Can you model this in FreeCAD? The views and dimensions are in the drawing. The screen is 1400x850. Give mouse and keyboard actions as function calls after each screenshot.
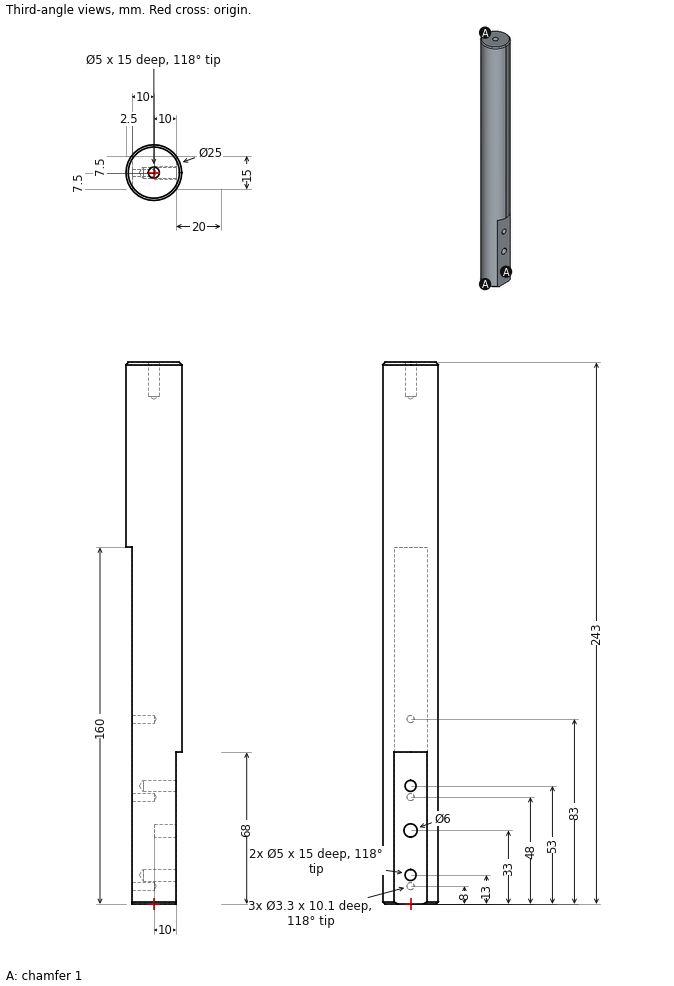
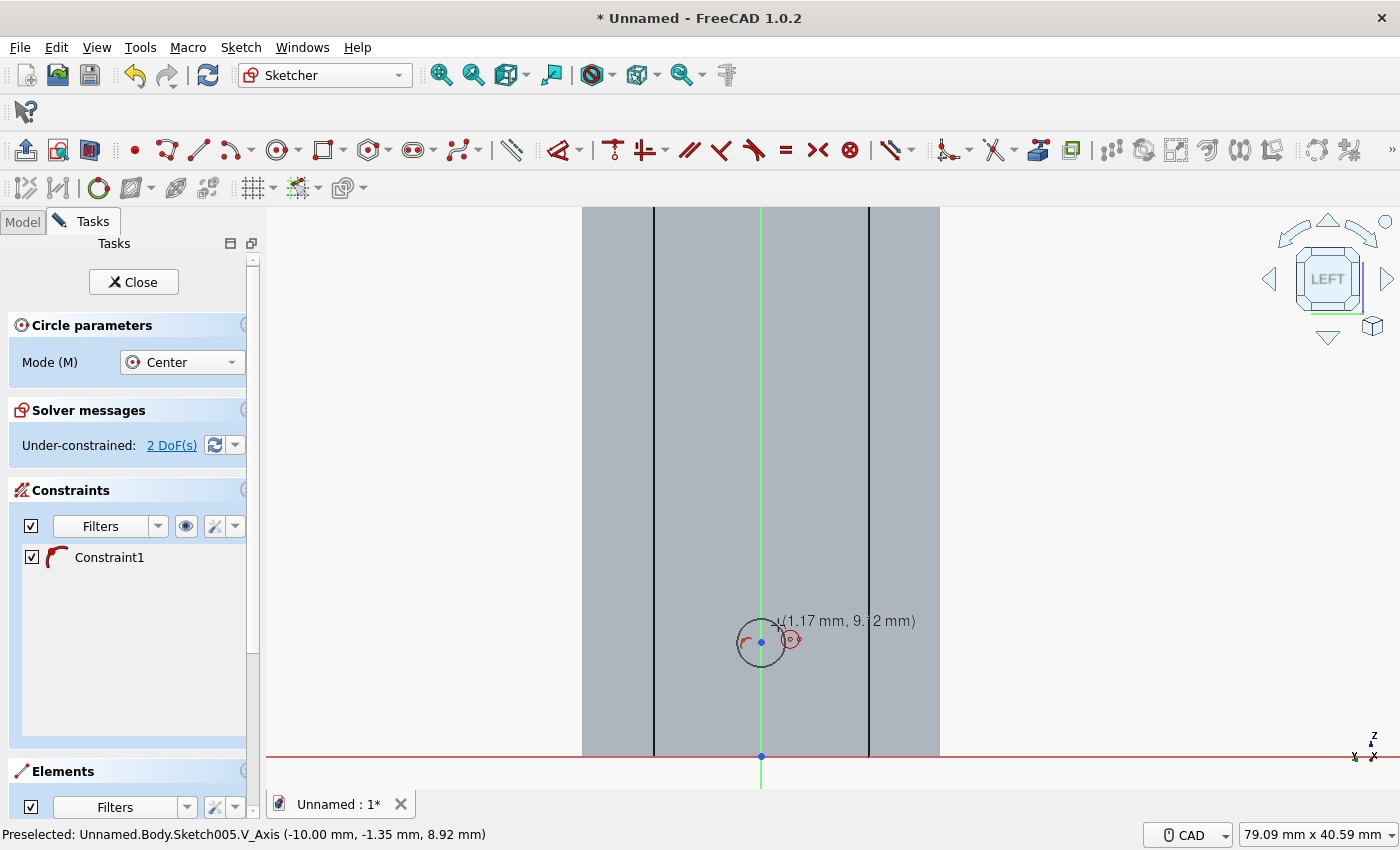
scroll(766, 648, down, 6)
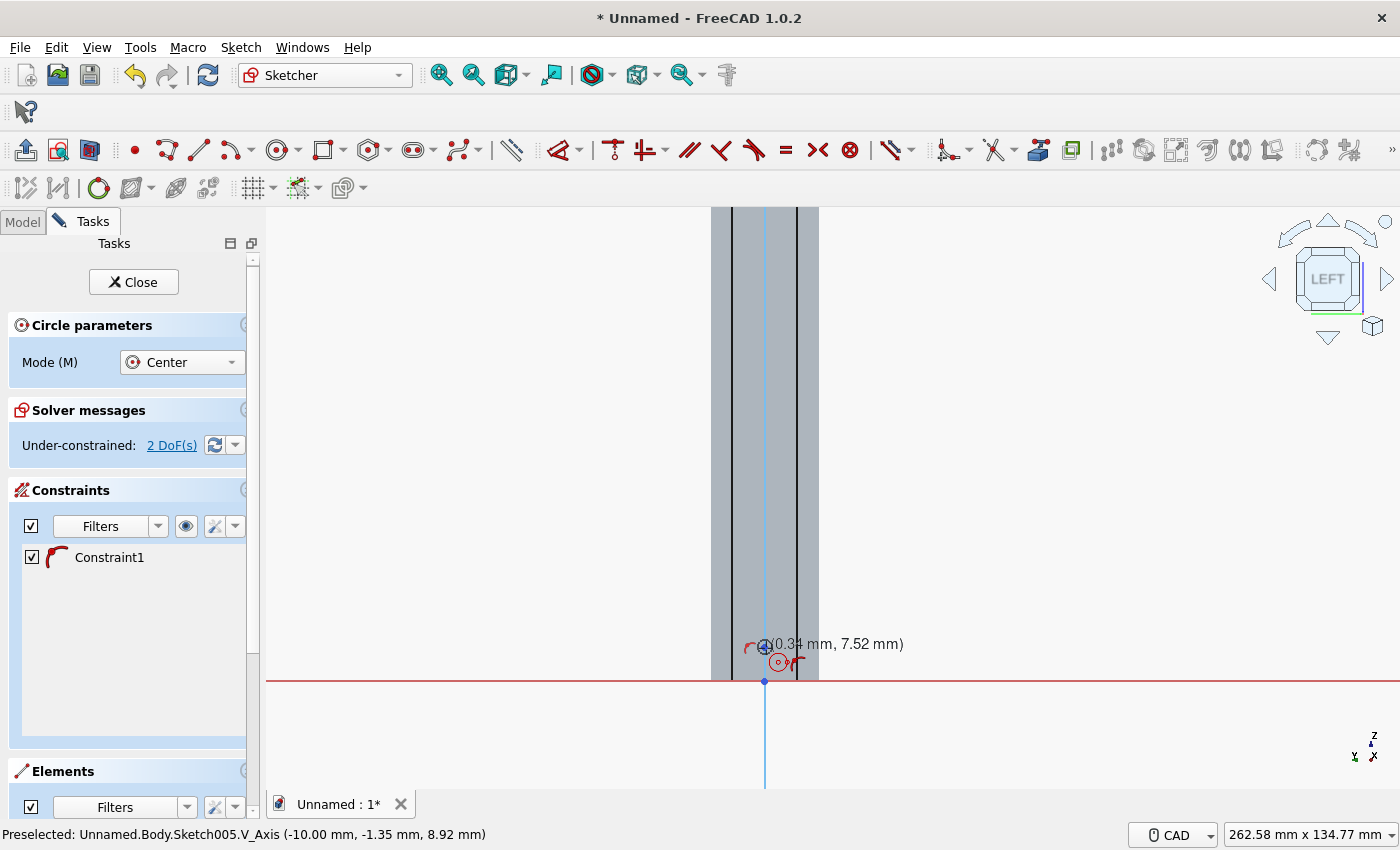
scroll(765, 323, up, 6)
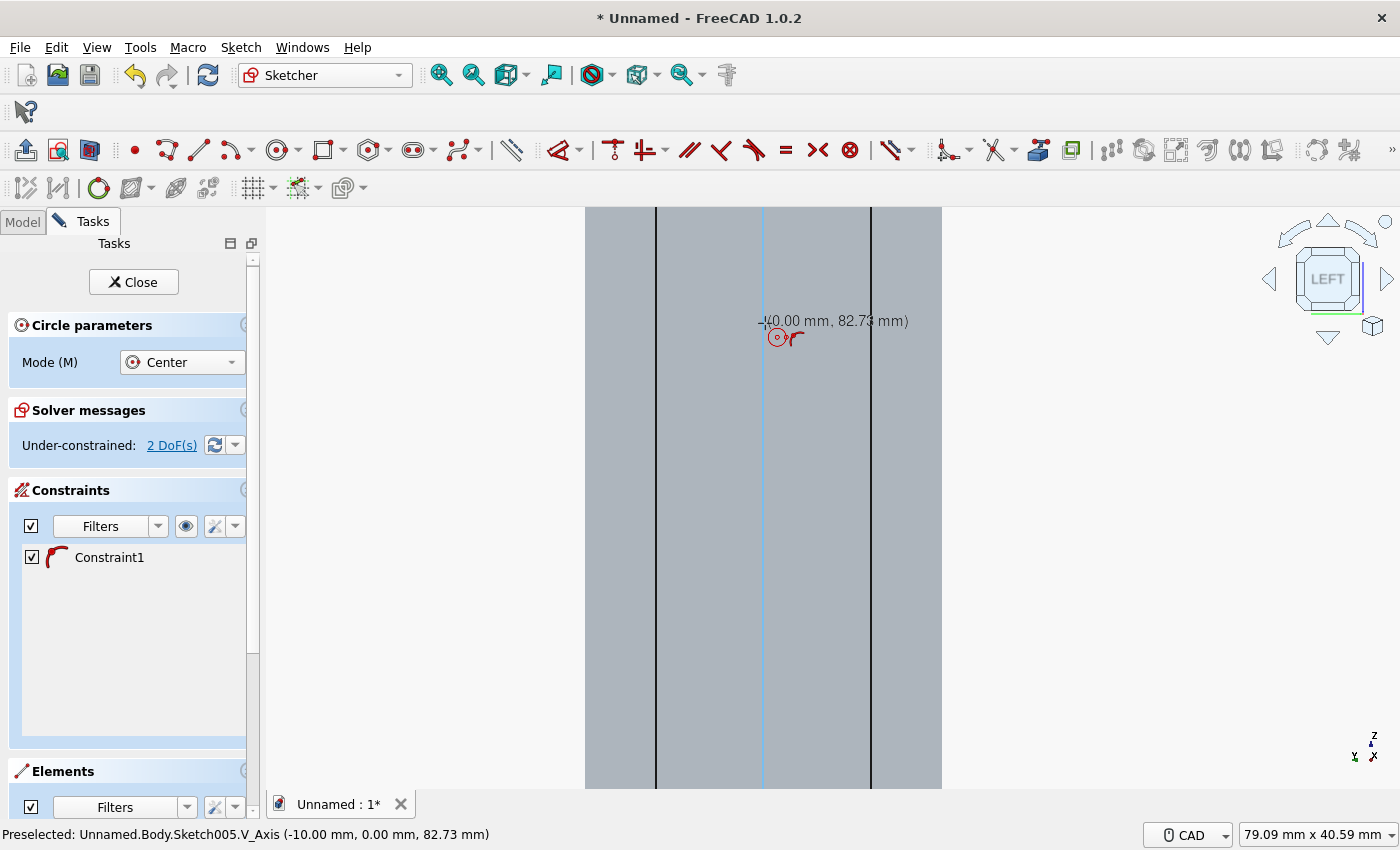
click(763, 322)
click(780, 305)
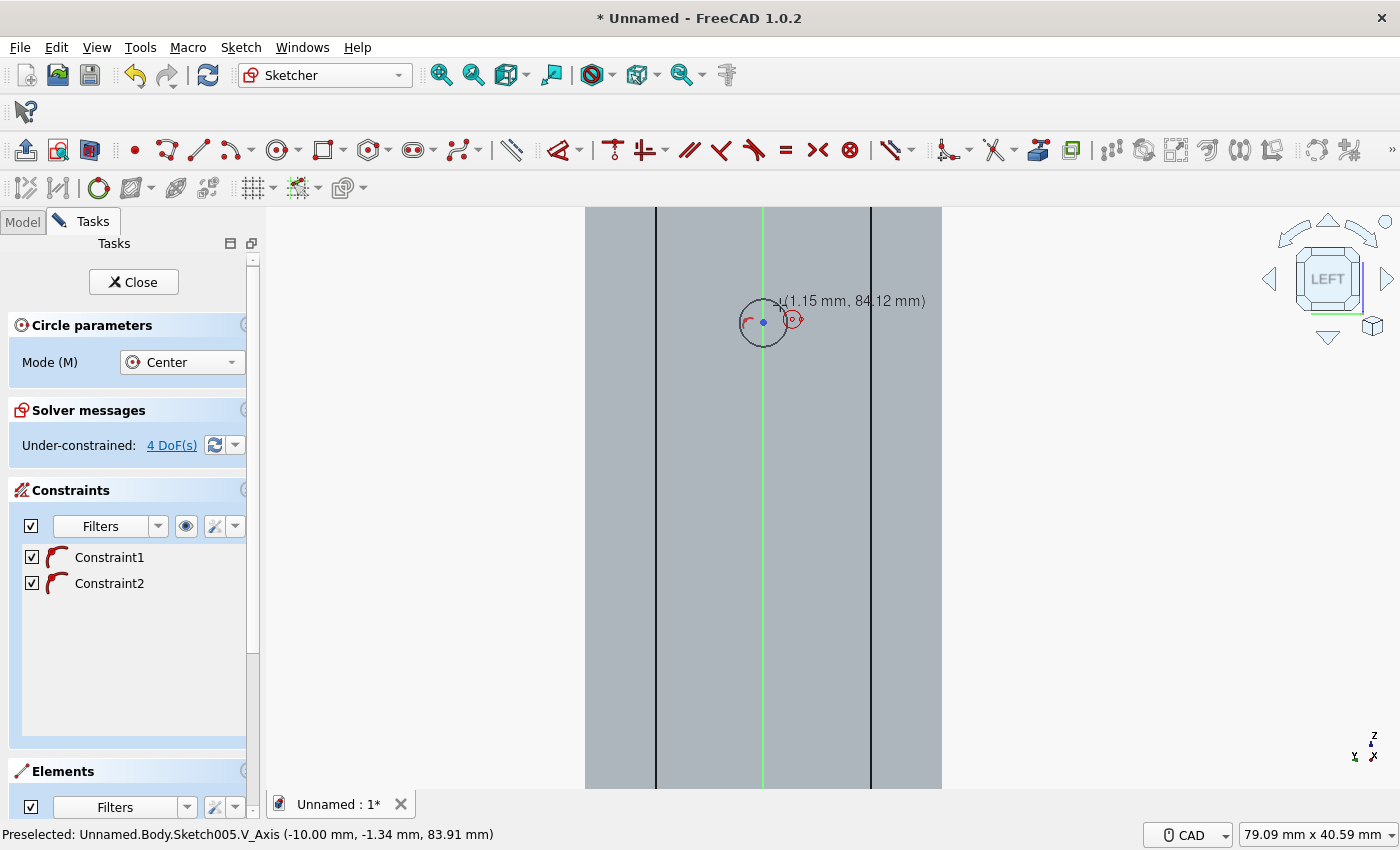
scroll(765, 322, down, 6)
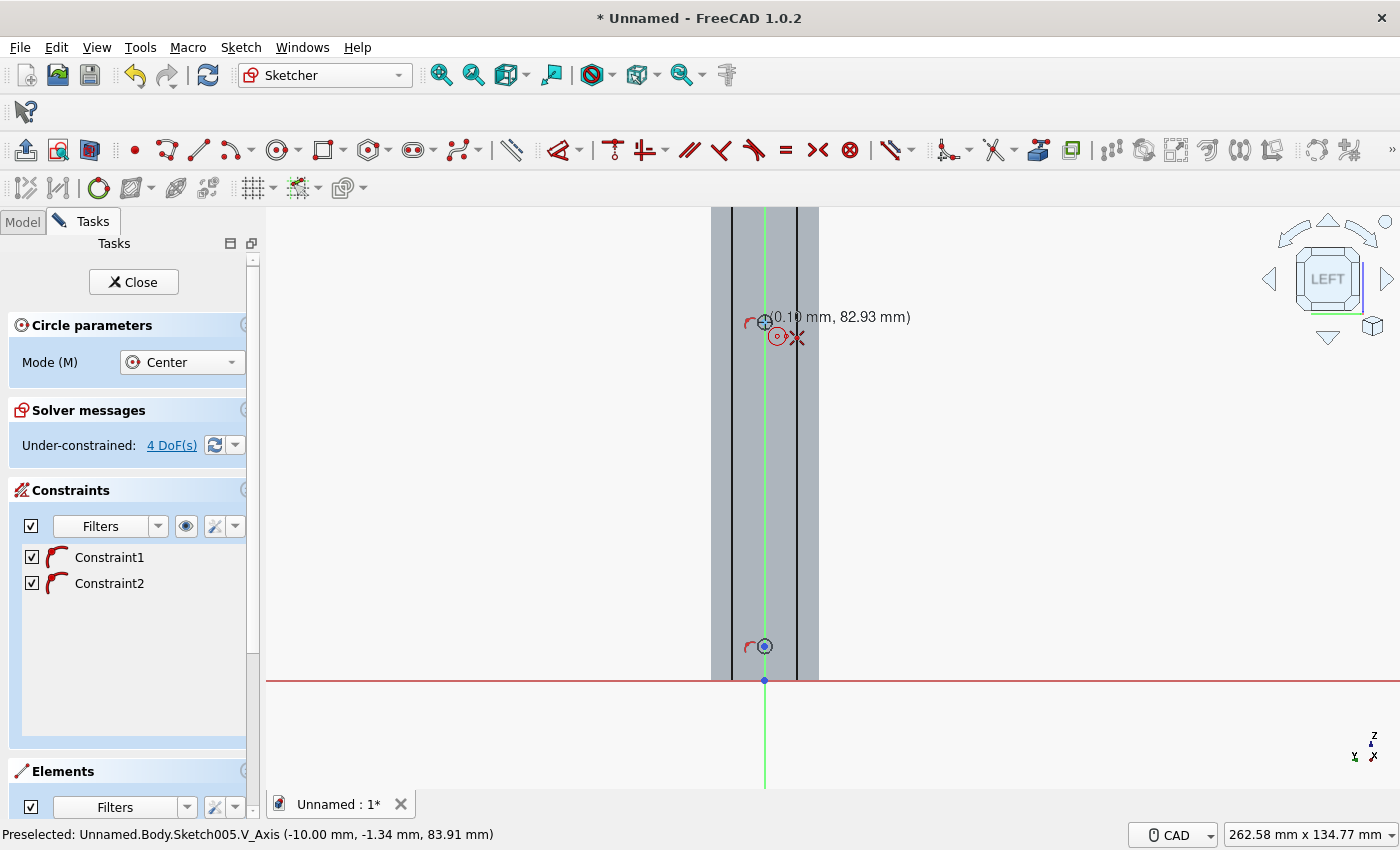
scroll(765, 473, up, 6)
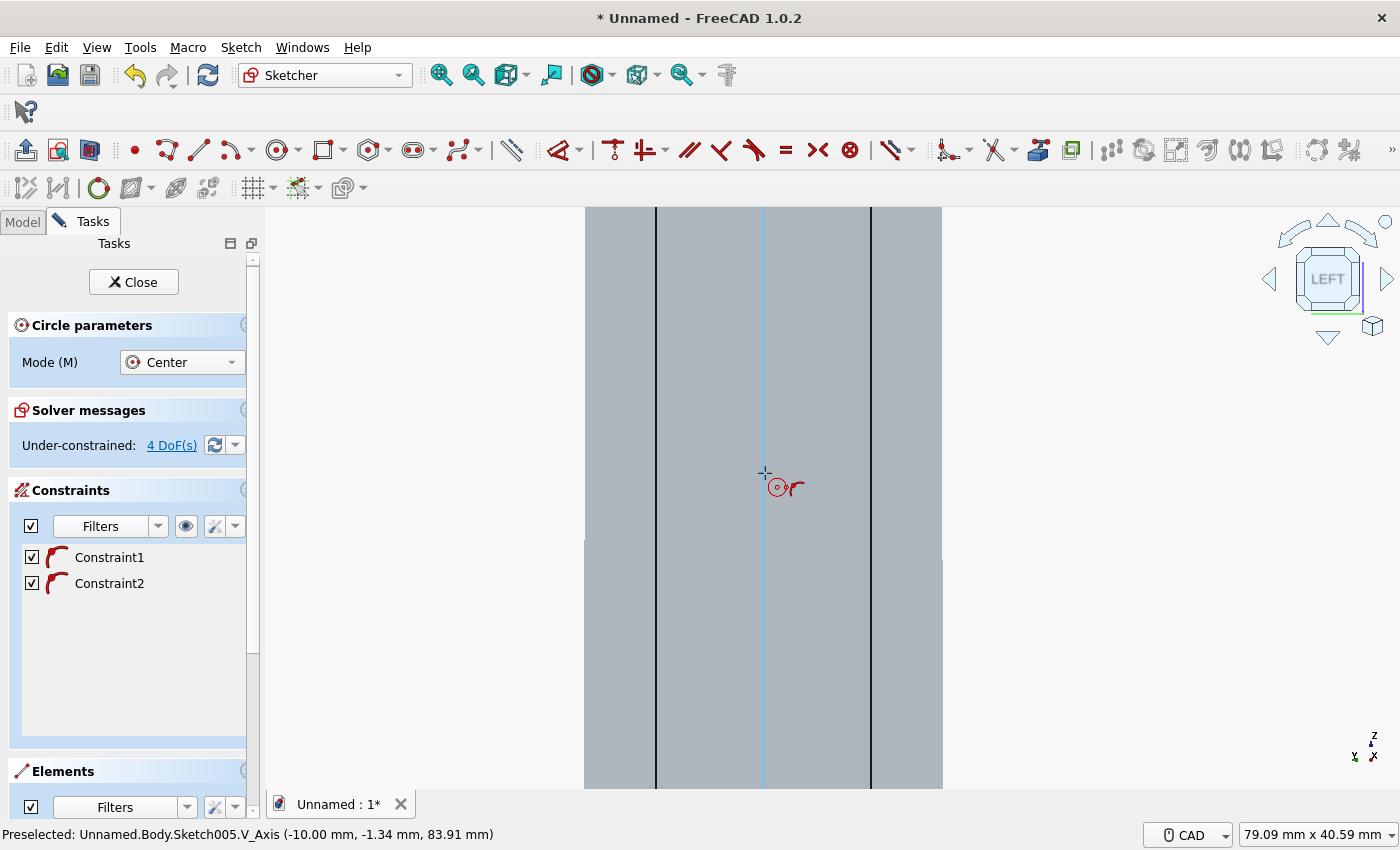
click(763, 473)
click(780, 456)
key(Escape)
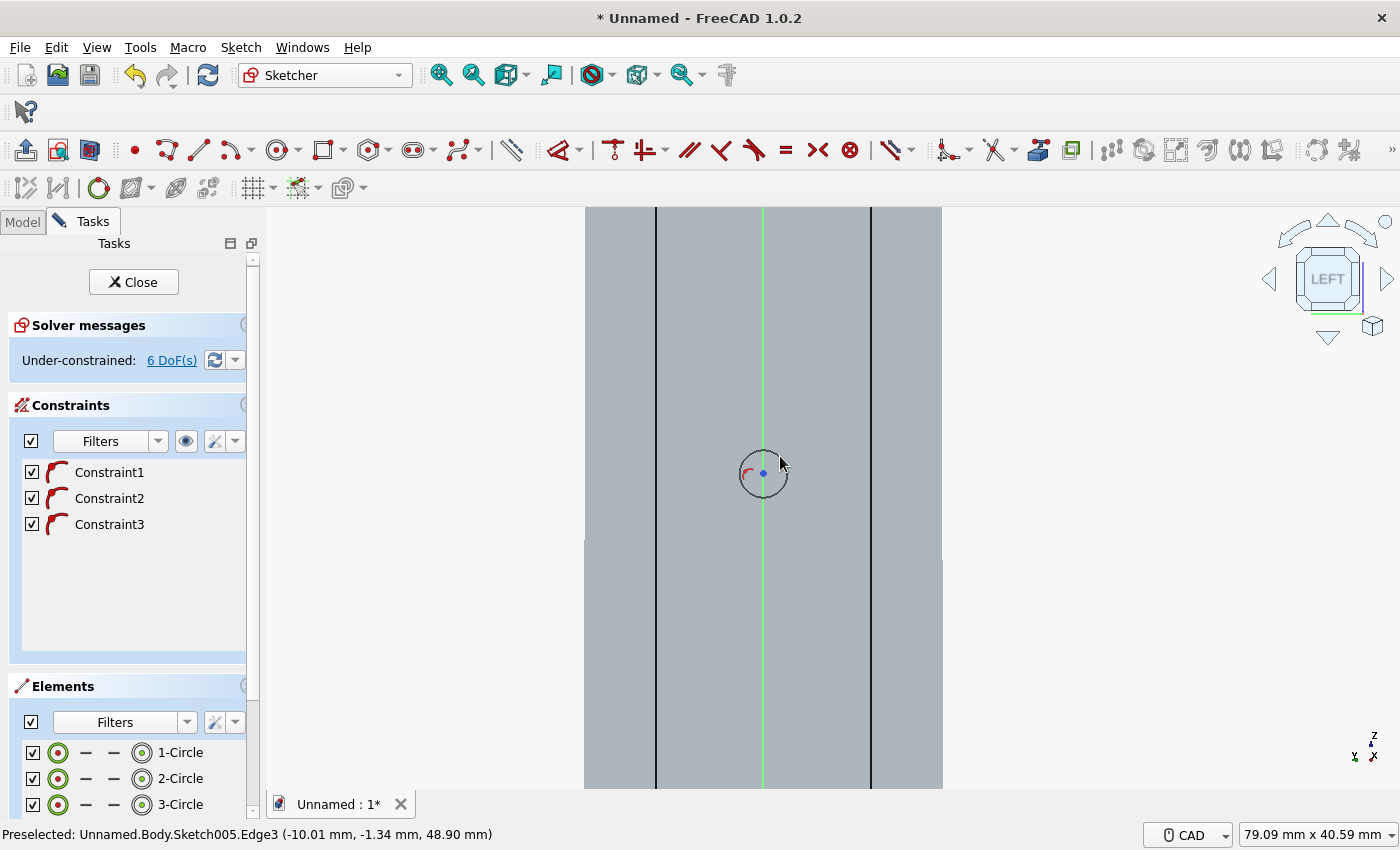
scroll(765, 474, down, 6)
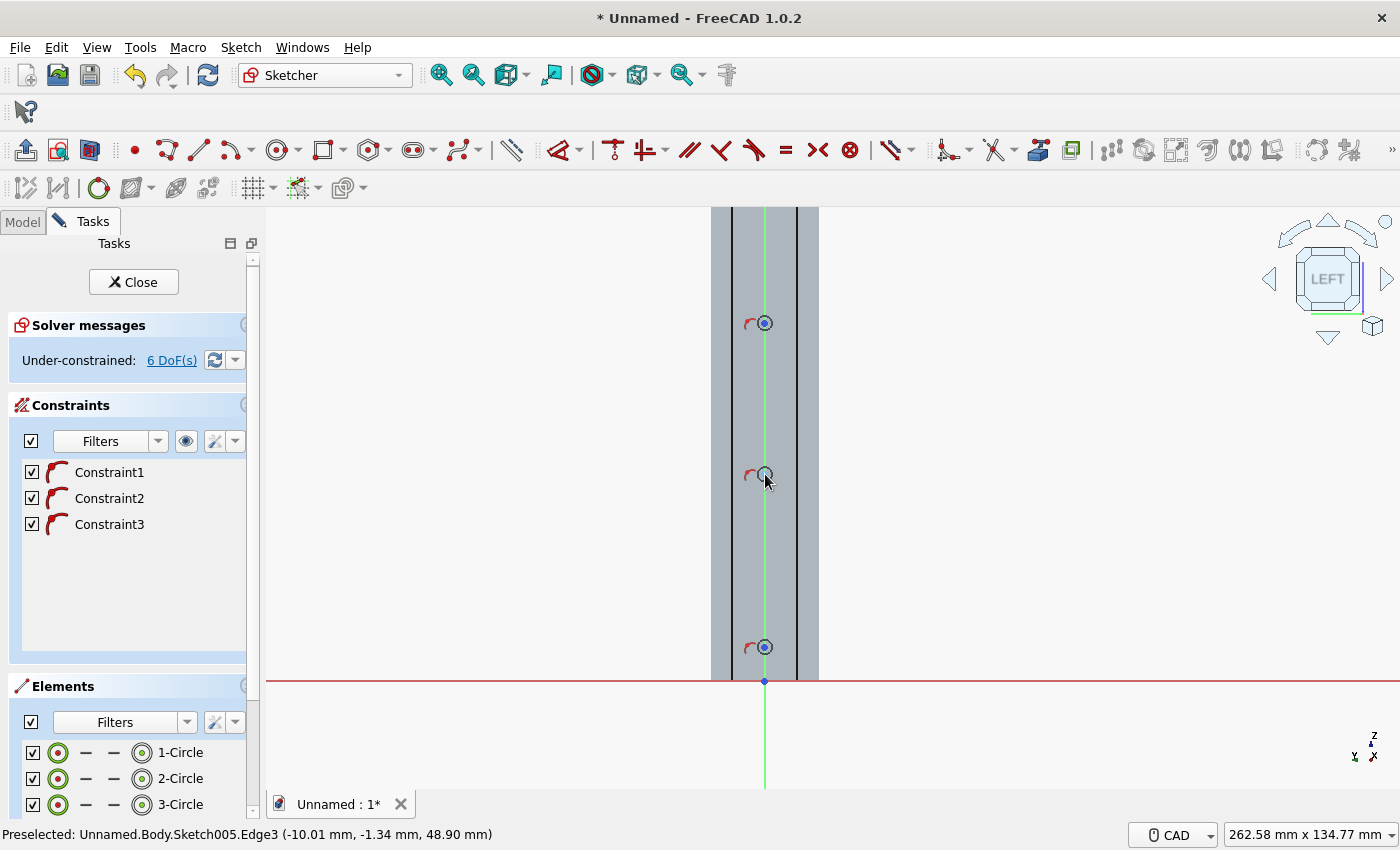
scroll(770, 642, up, 6)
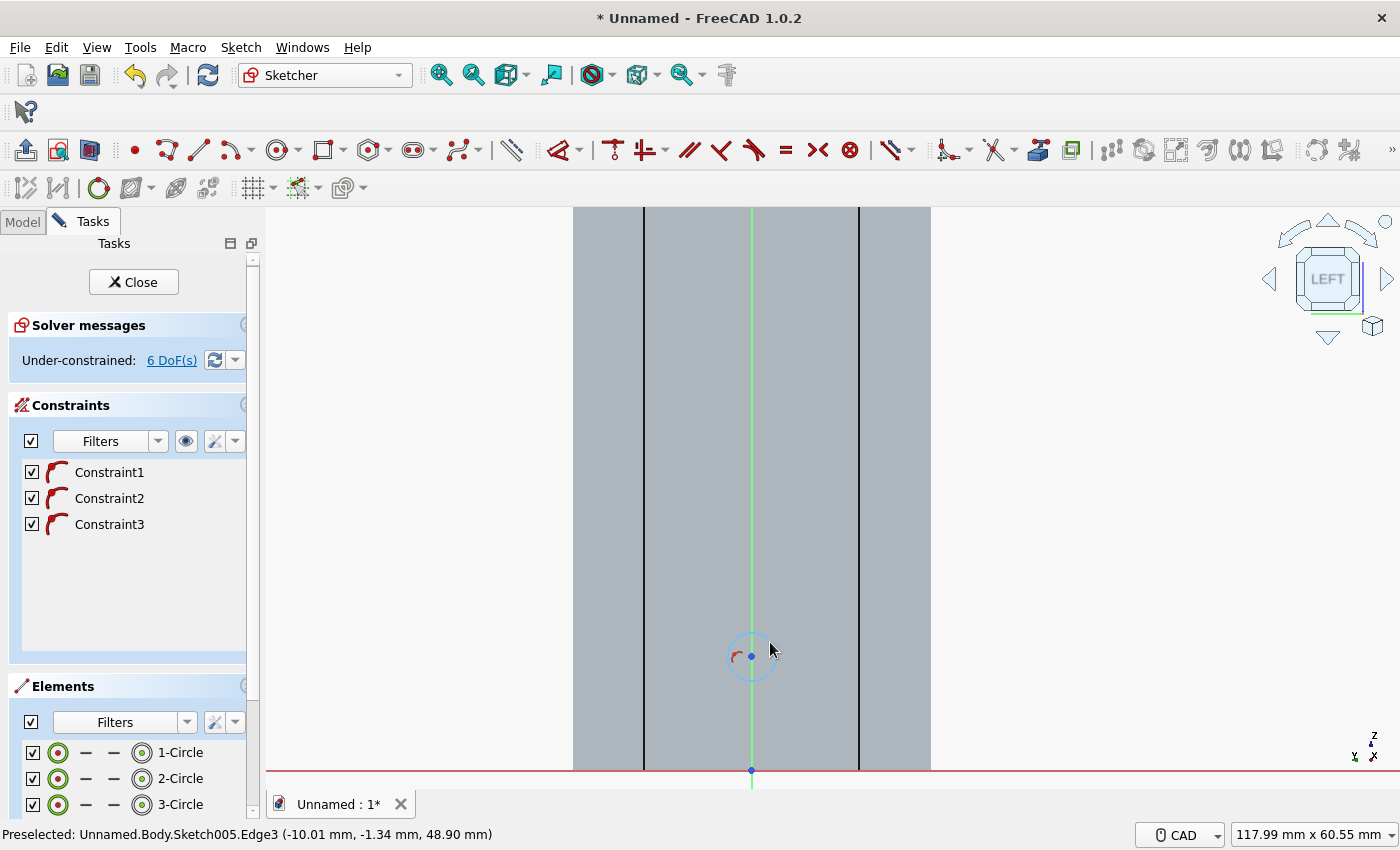
click(769, 640)